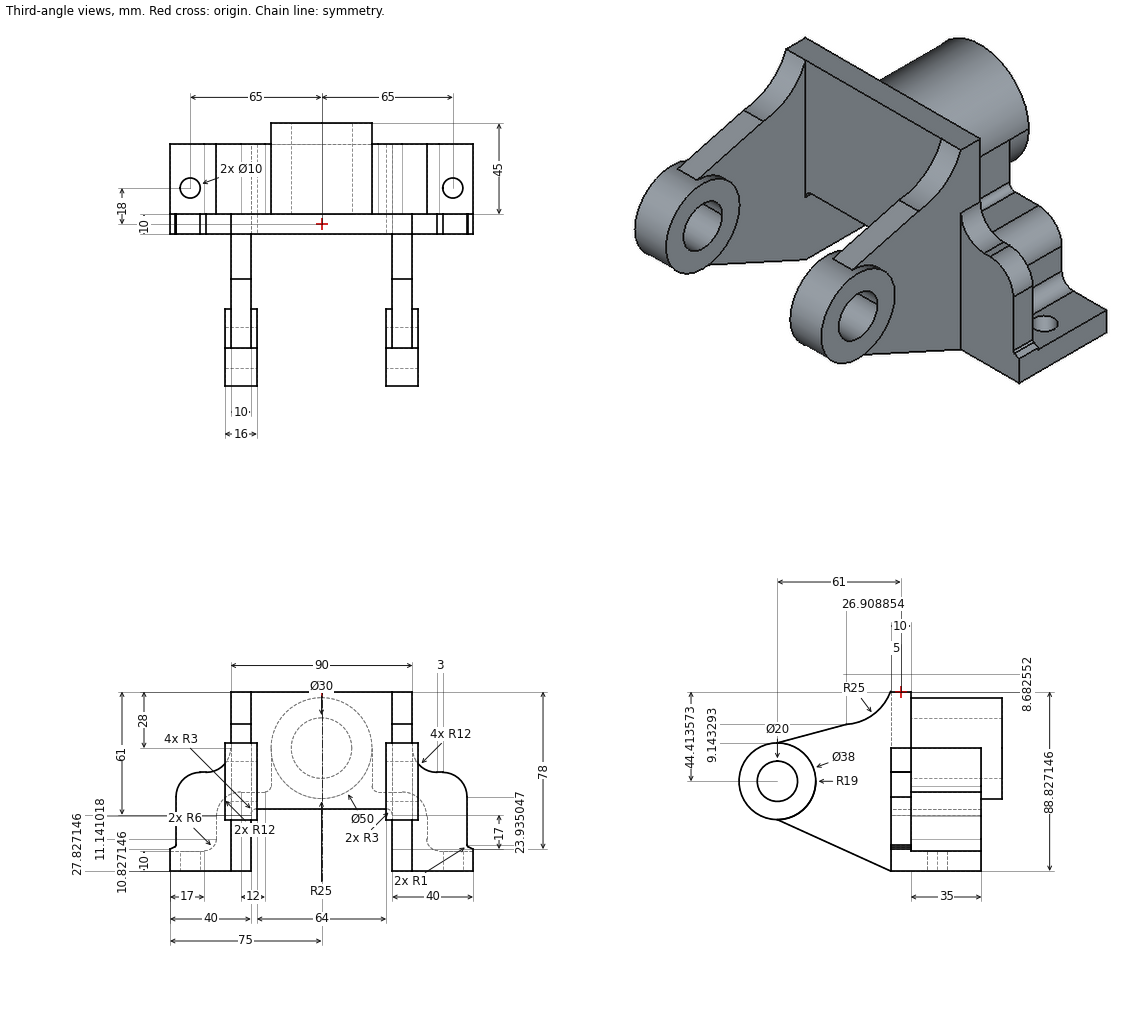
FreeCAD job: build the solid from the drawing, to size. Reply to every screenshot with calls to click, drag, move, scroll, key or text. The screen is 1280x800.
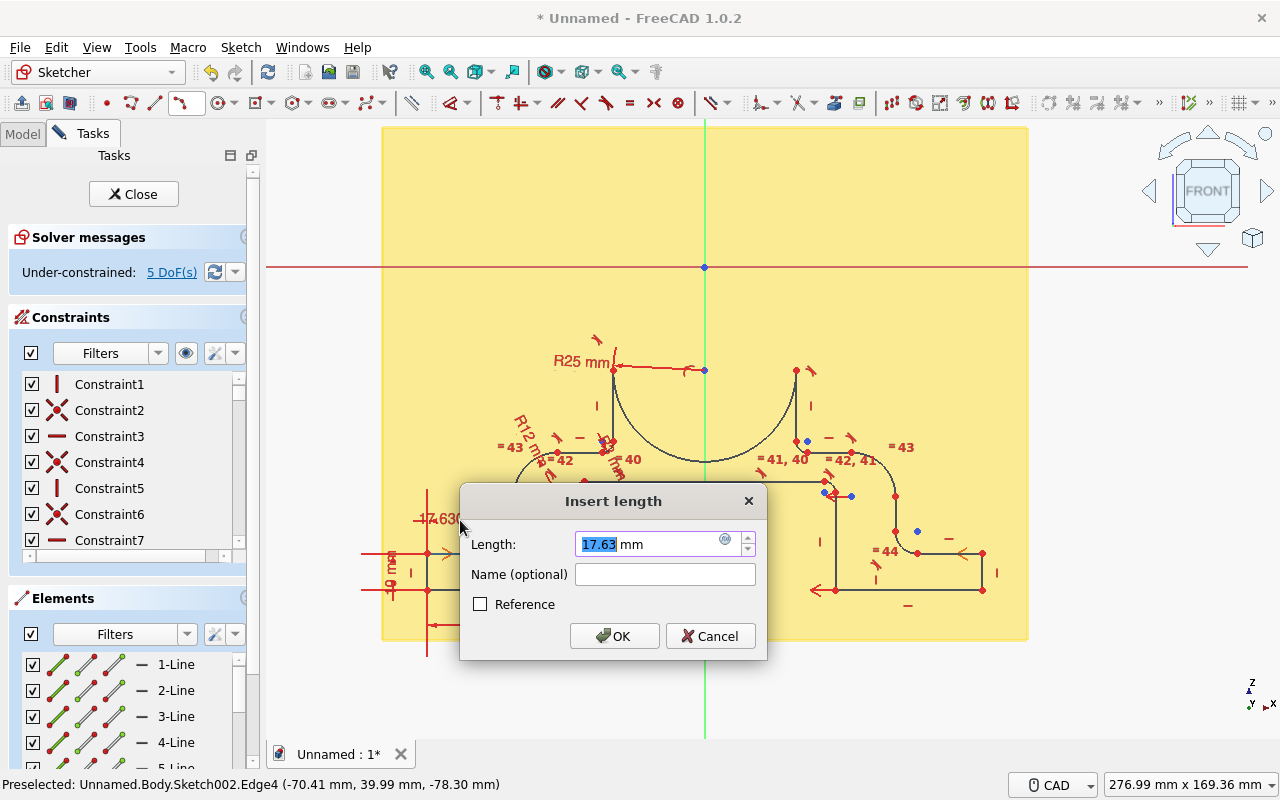
text(17)
key(Return)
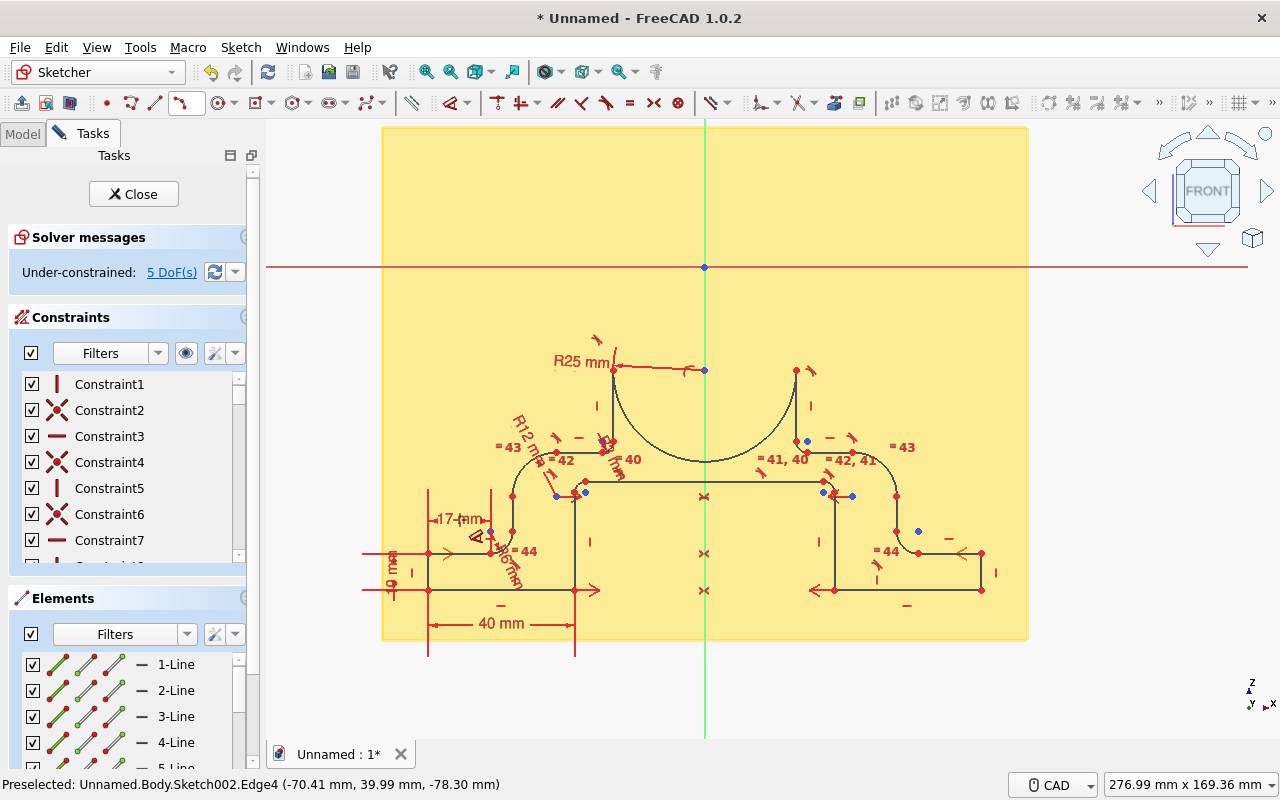
click(570, 453)
click(590, 511)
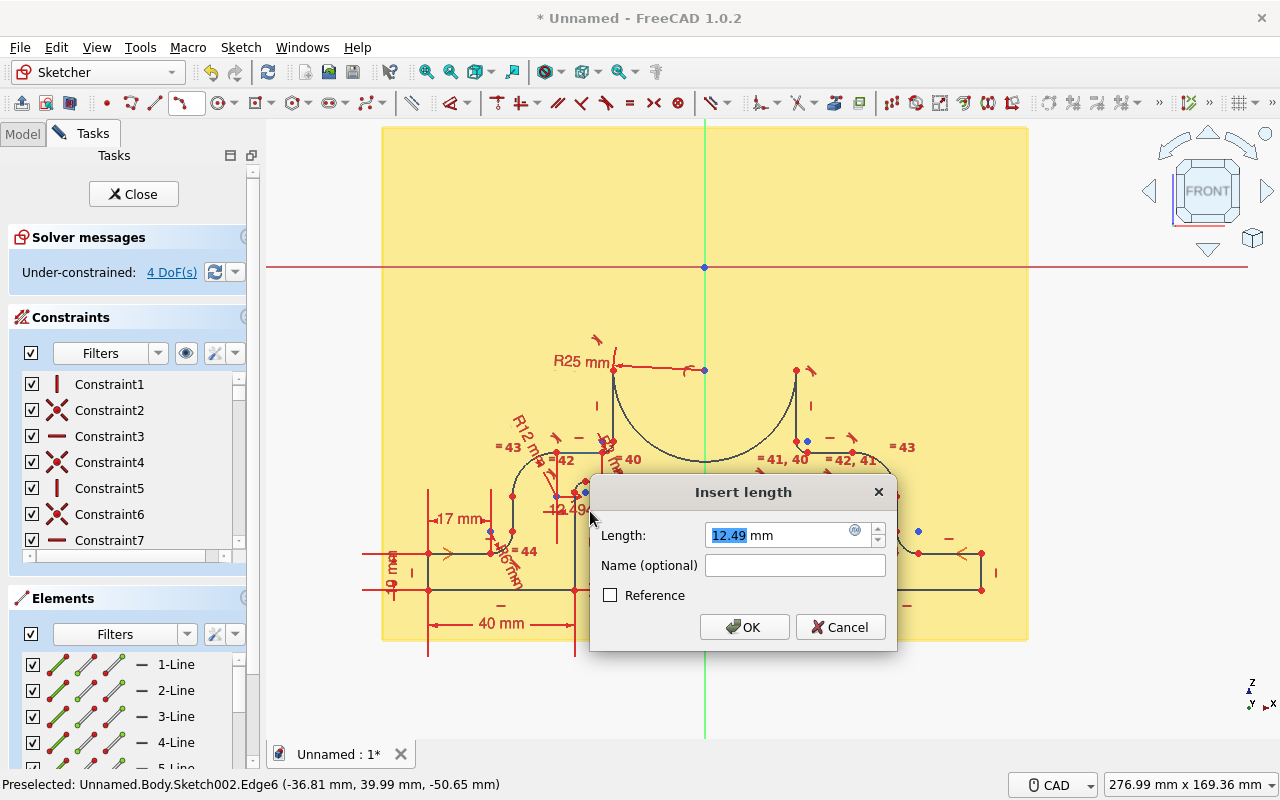
text(12)
key(Return)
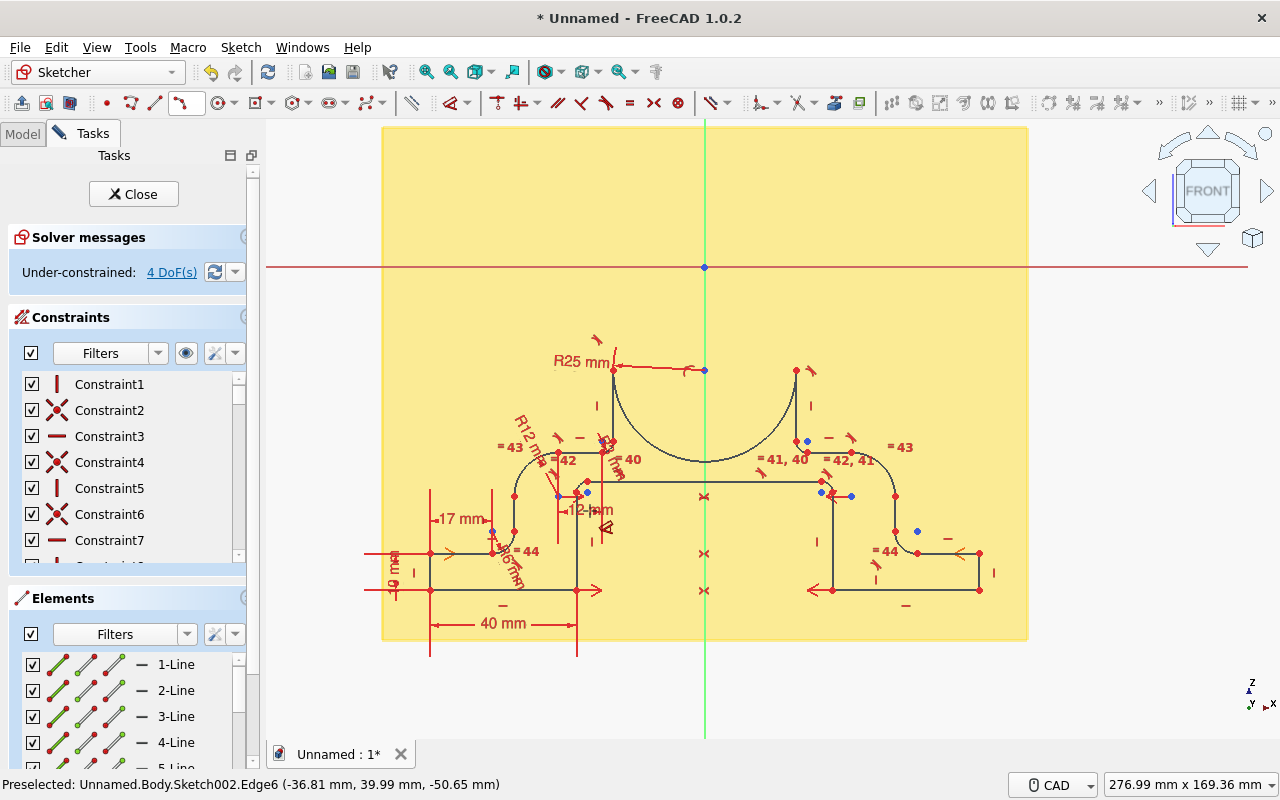
click(577, 493)
click(543, 328)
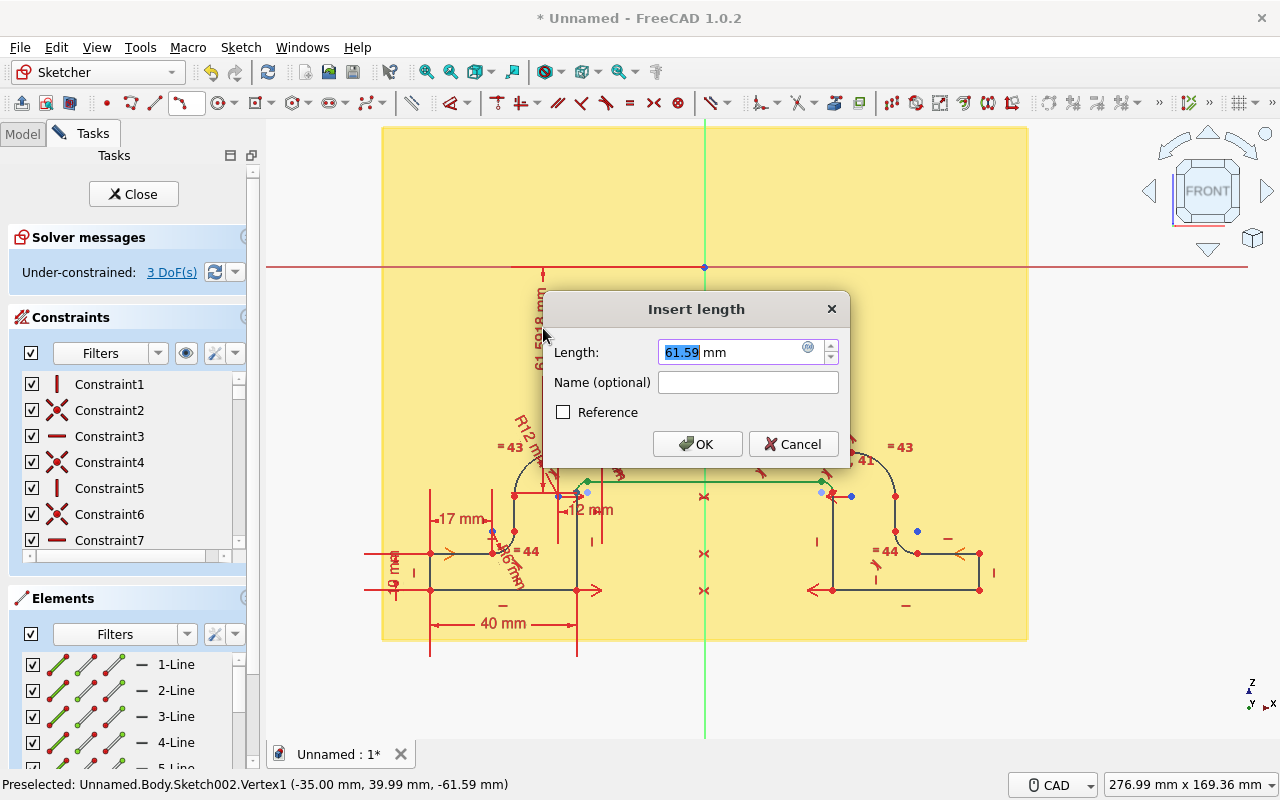
text(61)
key(Return)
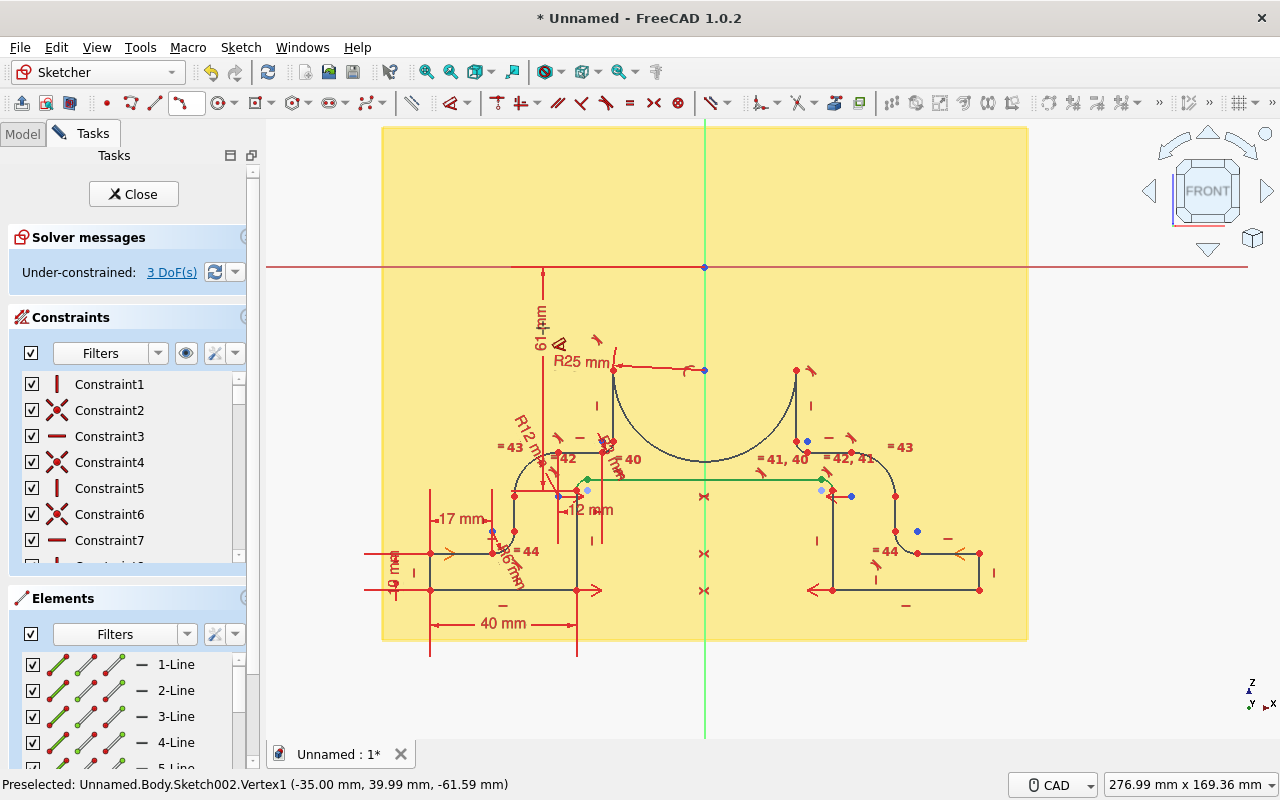
click(613, 370)
click(579, 295)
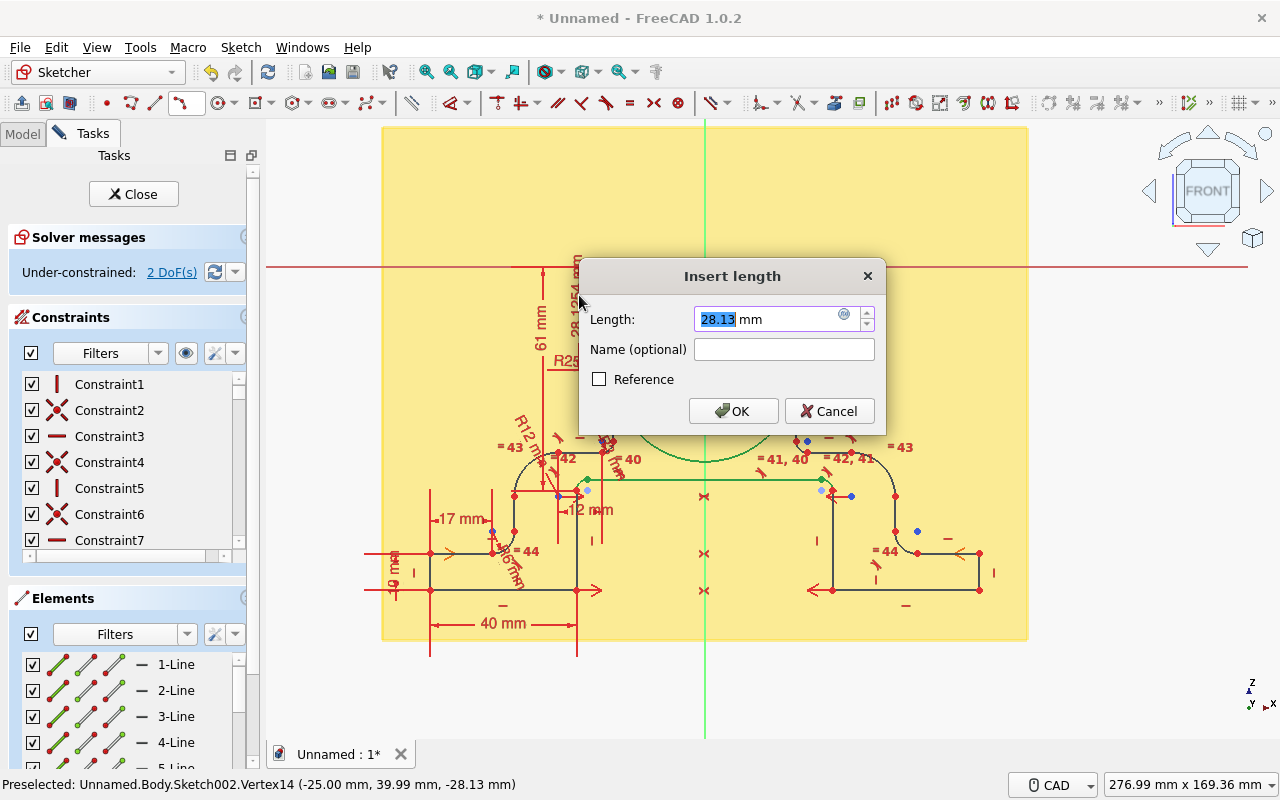
text(28)
key(Return)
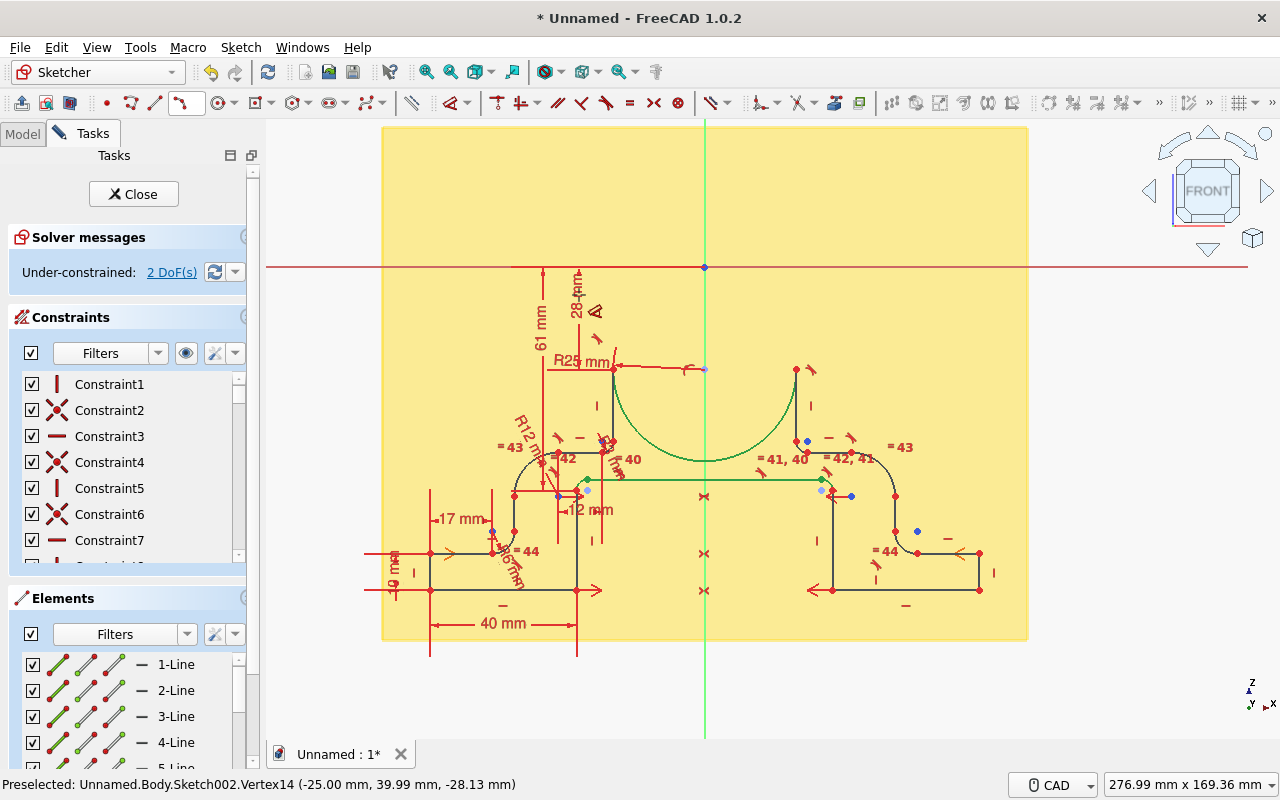
click(577, 520)
click(543, 540)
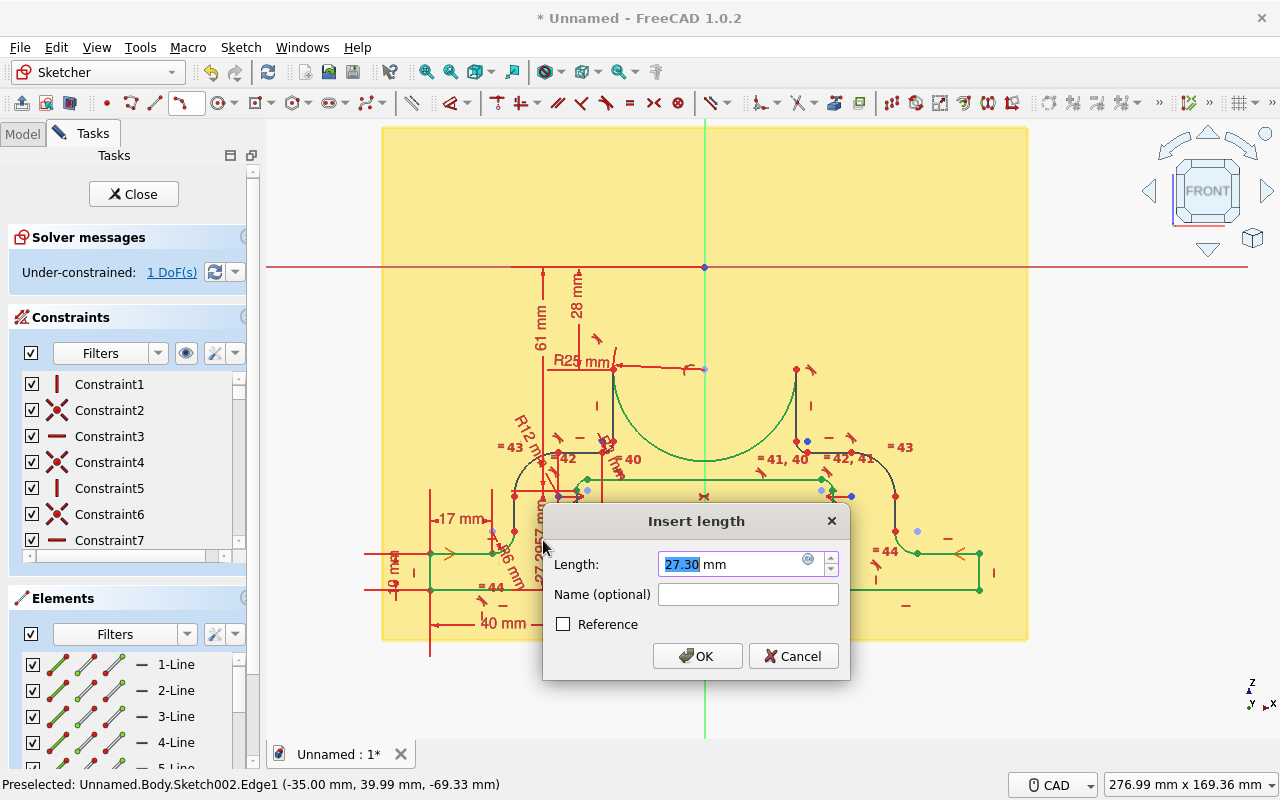
text(27.827146)
key(Return)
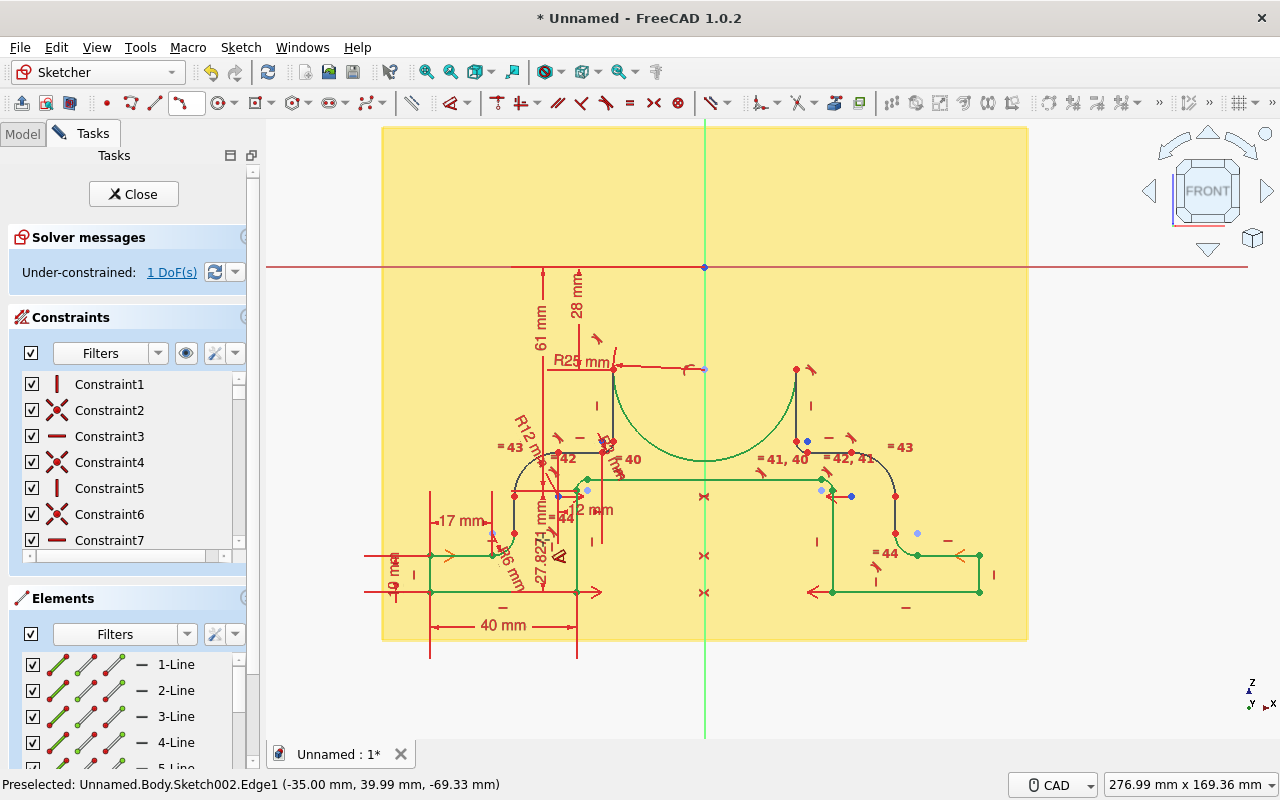
scroll(514, 523, up, 2)